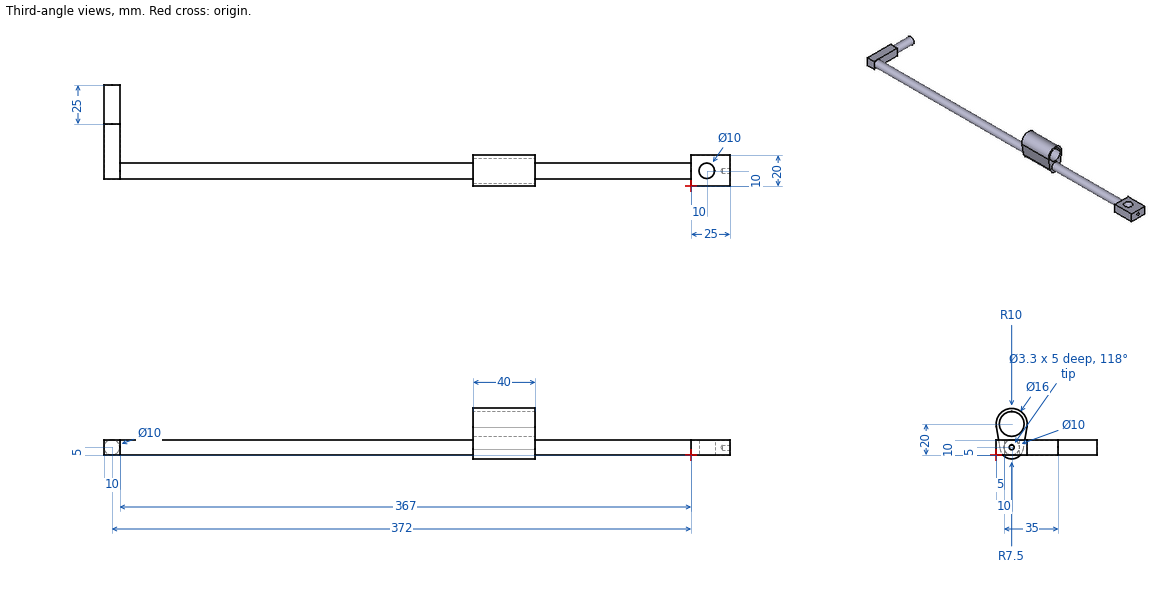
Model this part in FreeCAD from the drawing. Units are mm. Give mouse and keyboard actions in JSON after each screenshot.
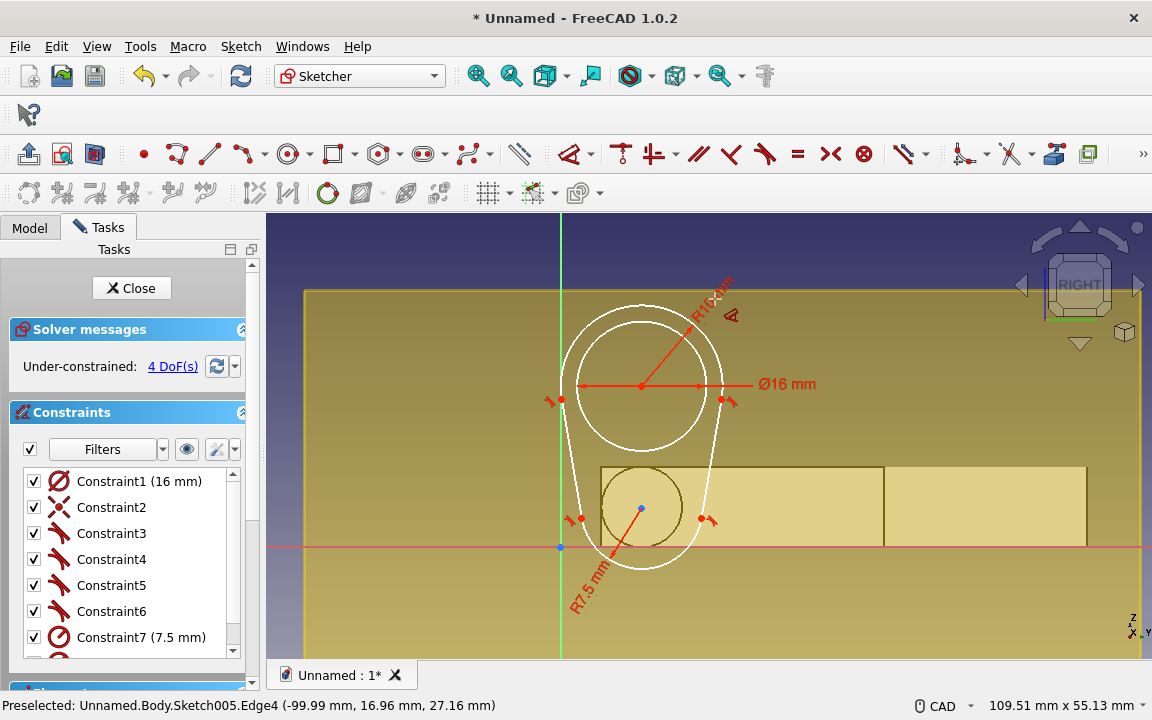
{"action": "left_click", "coordinate": [642, 508]}
{"action": "left_click", "coordinate": [527, 528]}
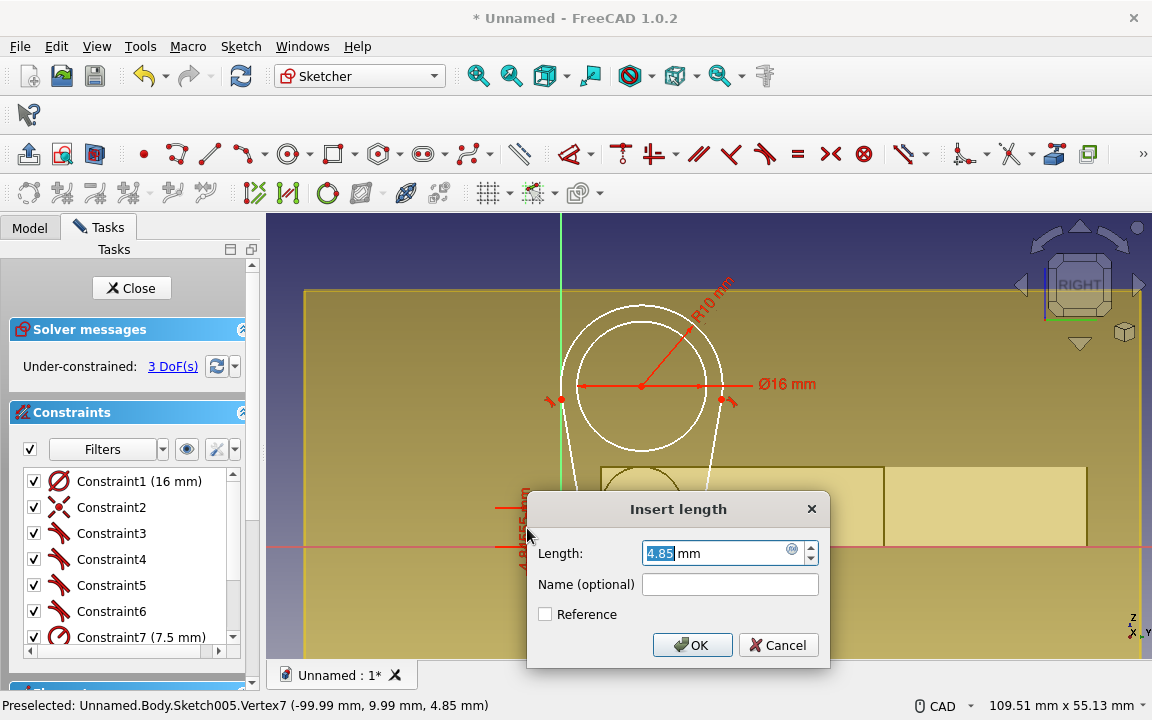
{"action": "type", "text": "5"}
{"action": "key", "text": "Return"}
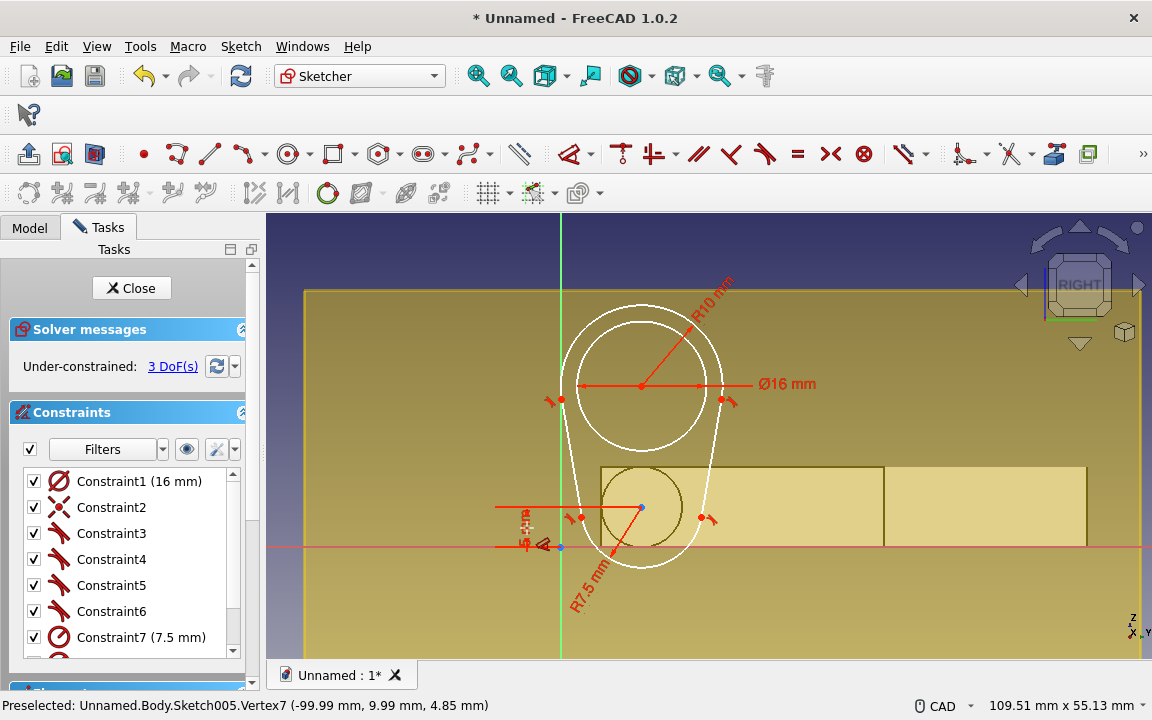
{"action": "left_click", "coordinate": [642, 386]}
{"action": "left_click", "coordinate": [620, 352]}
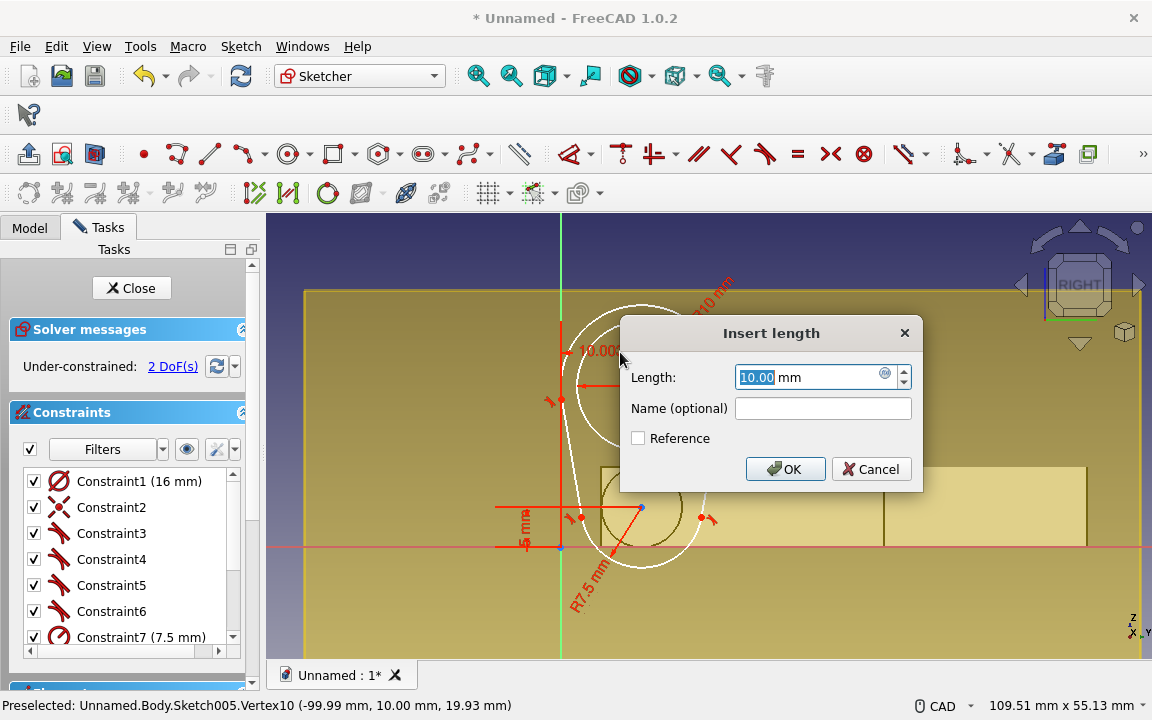
{"action": "type", "text": "10"}
{"action": "key", "text": "Return"}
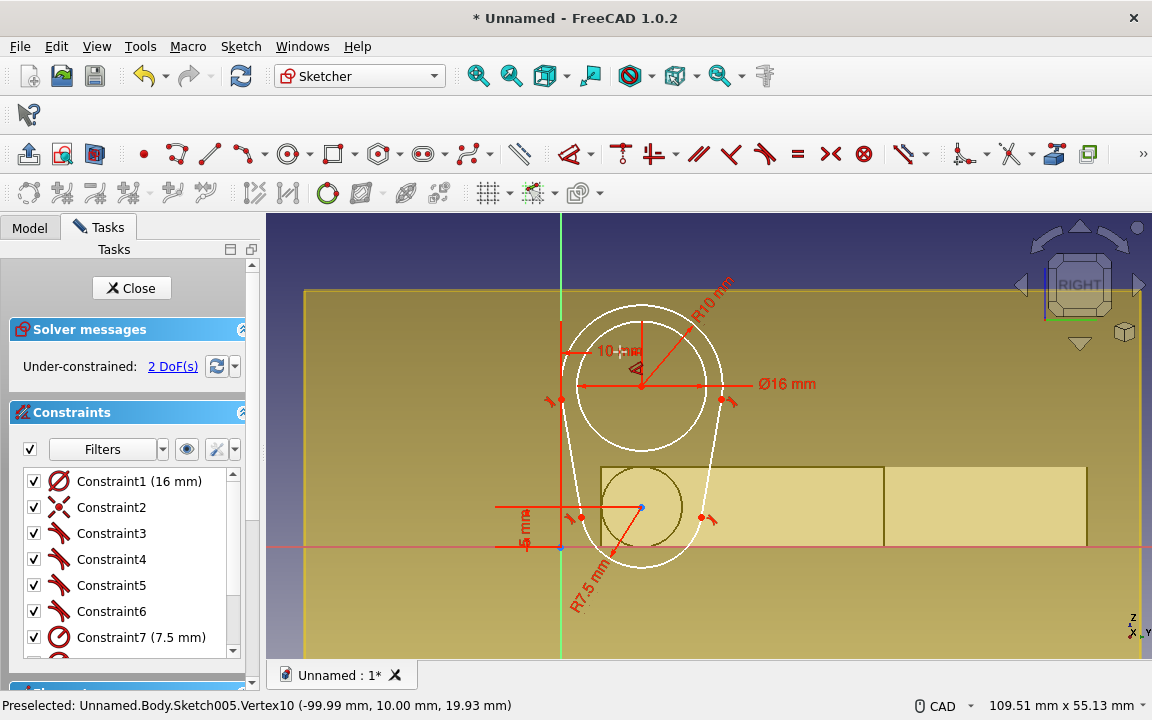
{"action": "left_click", "coordinate": [642, 386]}
{"action": "left_click", "coordinate": [527, 467]}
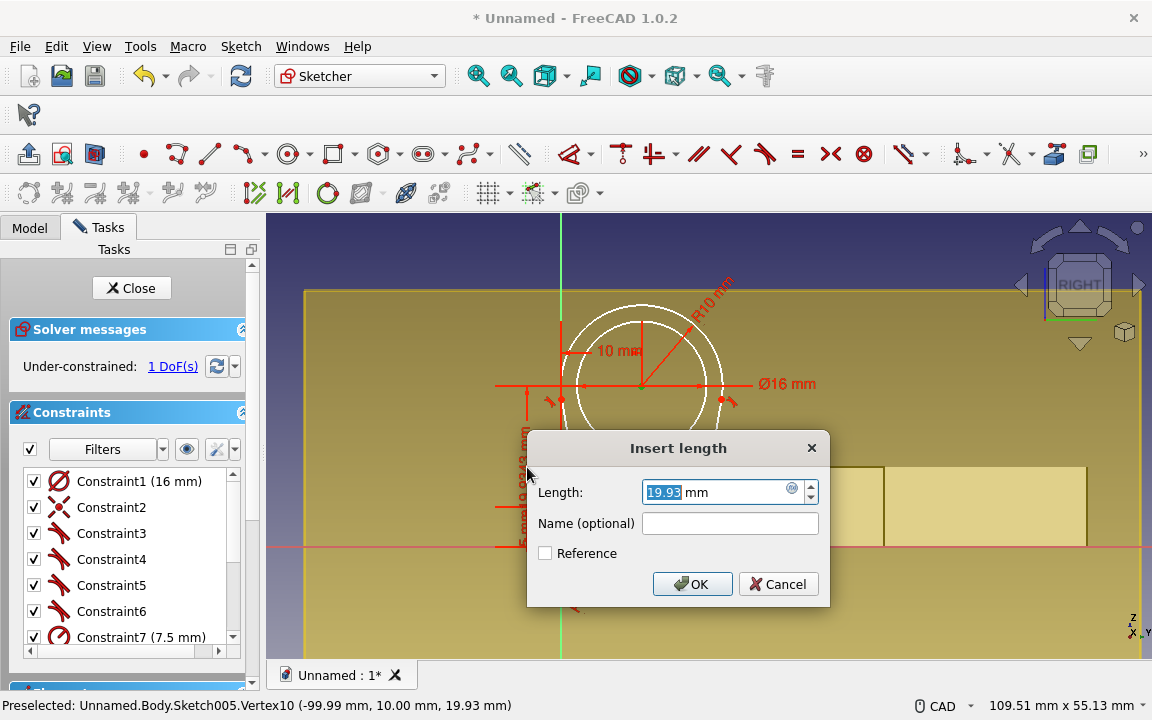
{"action": "type", "text": "20"}
{"action": "key", "text": "Return"}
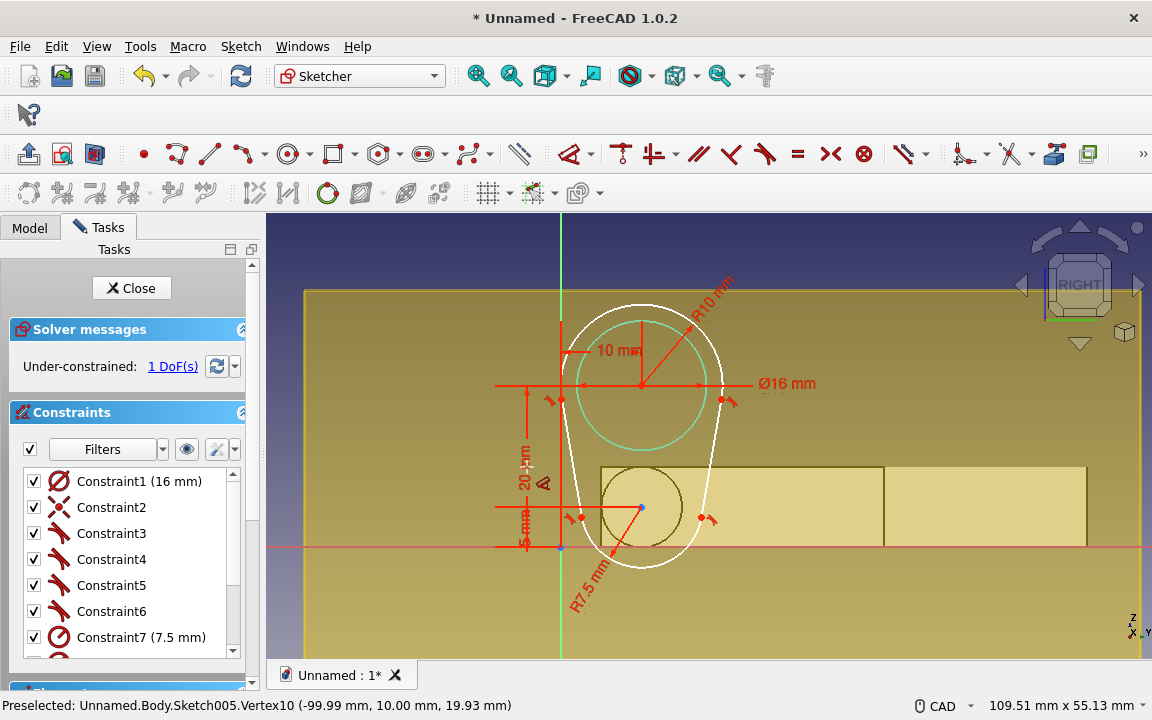
{"action": "left_click", "coordinate": [642, 507]}
{"action": "left_click", "coordinate": [601, 473]}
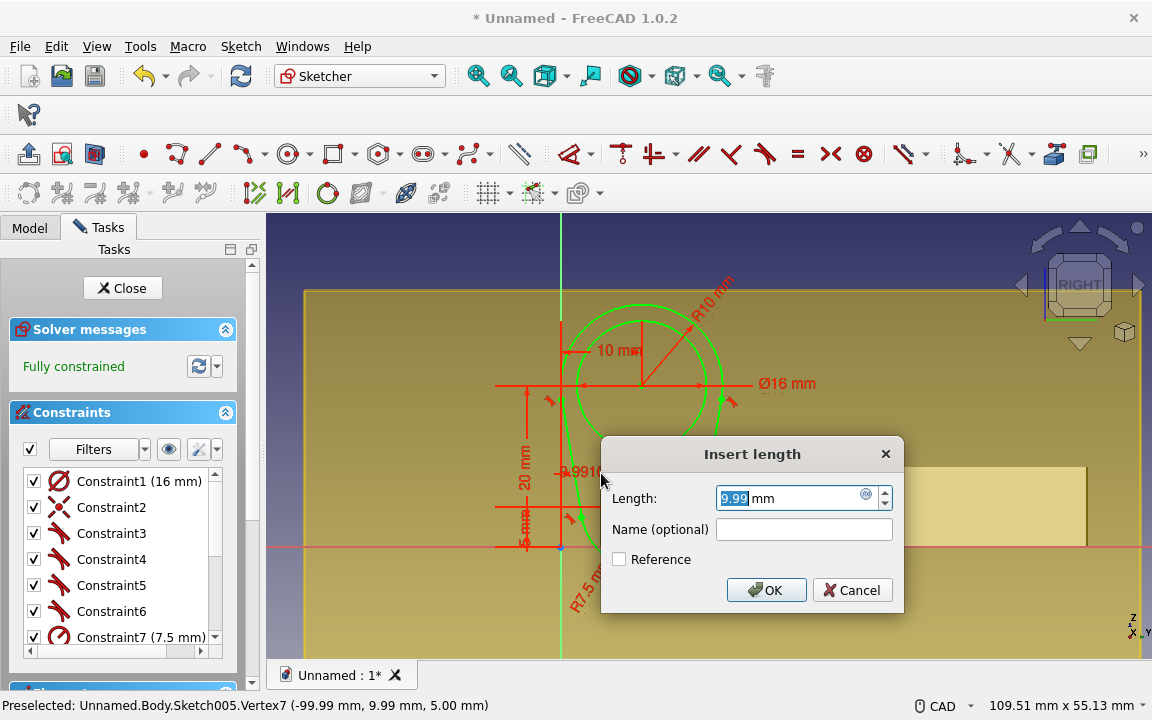
{"action": "type", "text": "10"}
{"action": "key", "text": "Return"}
{"action": "key", "text": "Escape"}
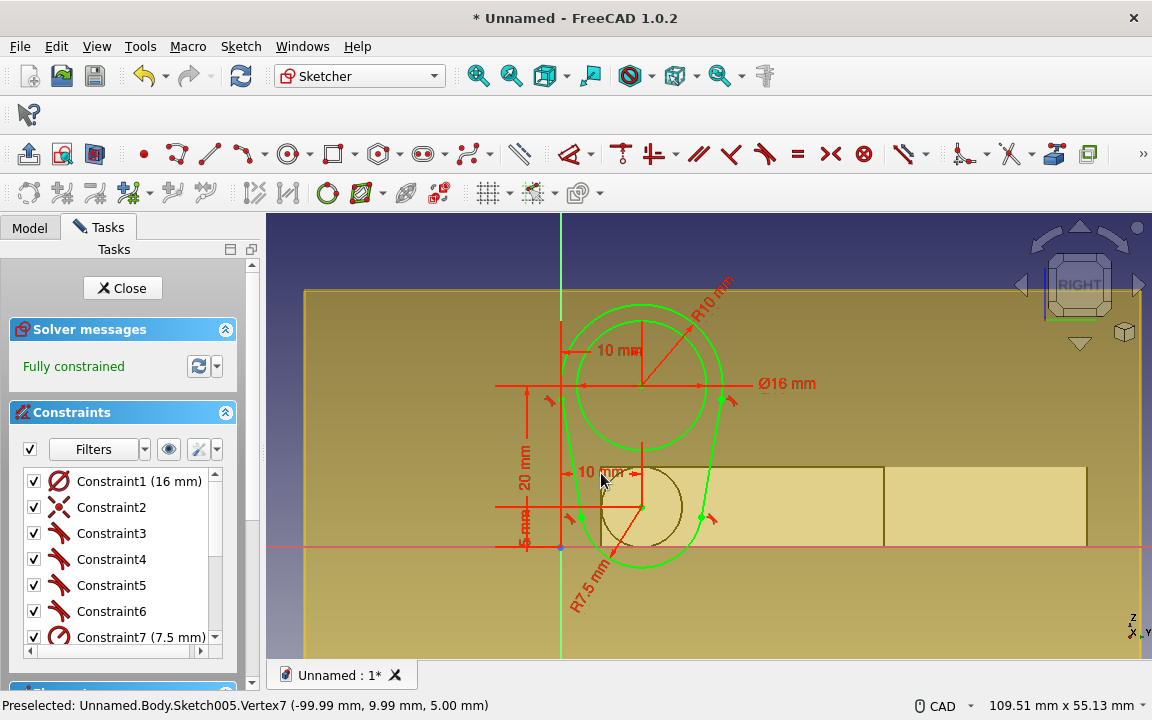
{"action": "left_click", "coordinate": [123, 288]}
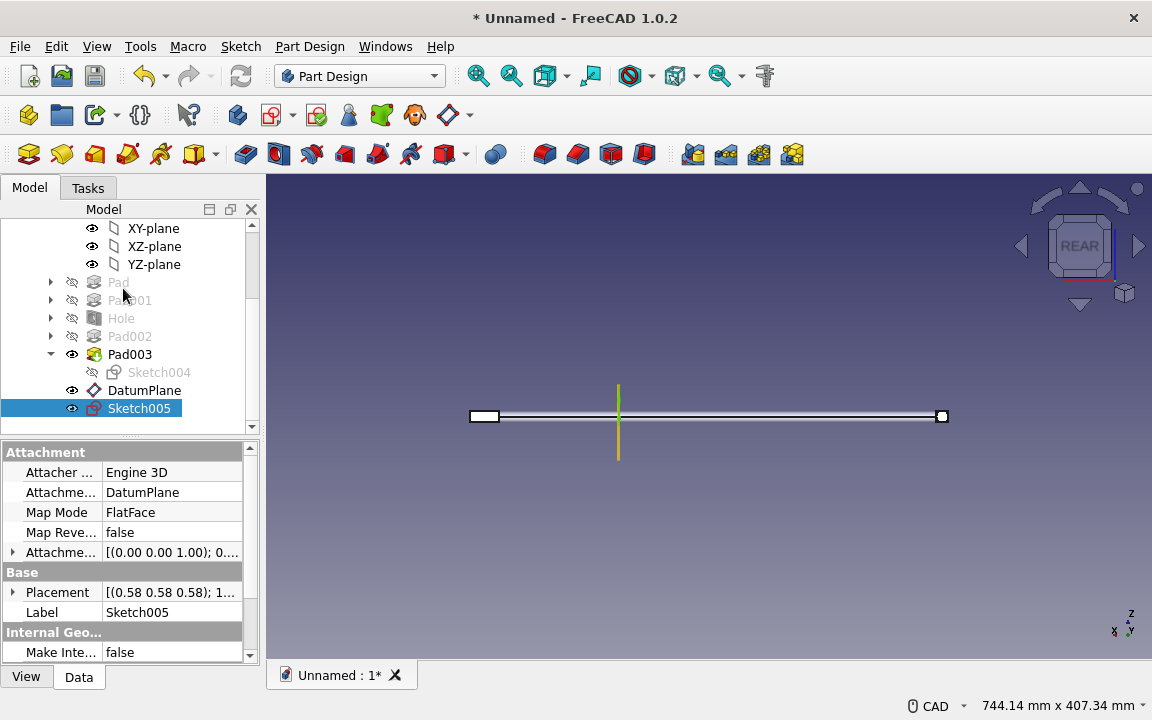
{"action": "left_click", "coordinate": [29, 154]}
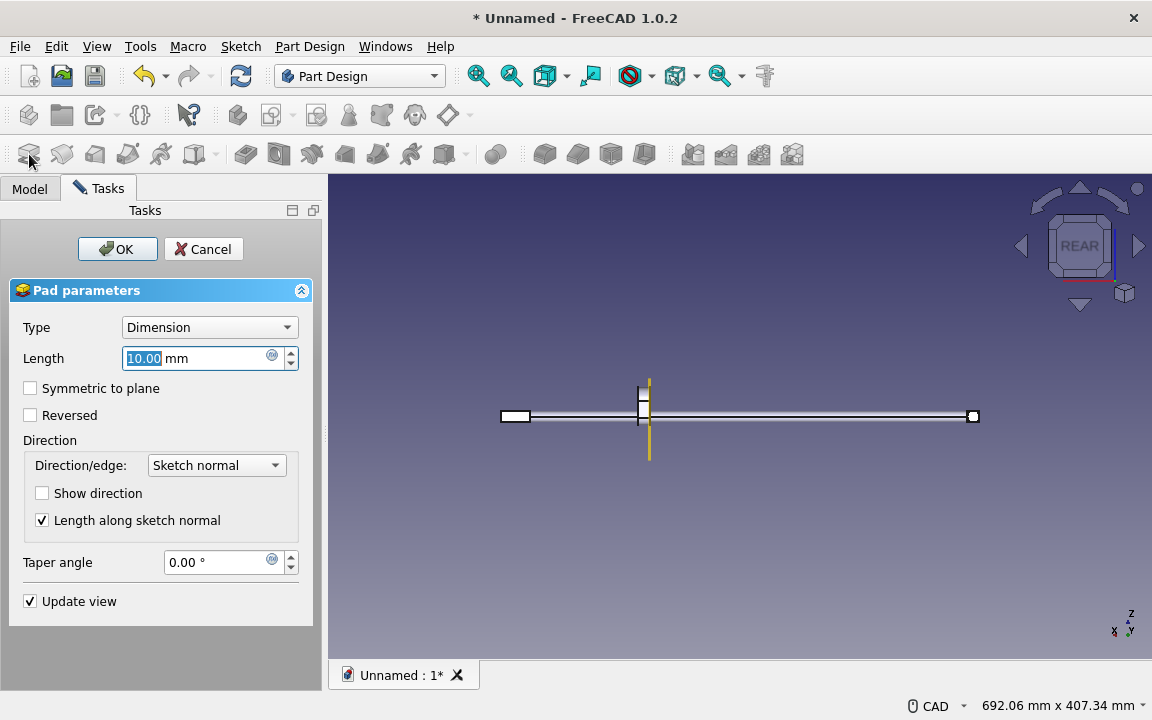
{"action": "type", "text": "40"}
{"action": "key", "text": "Tab"}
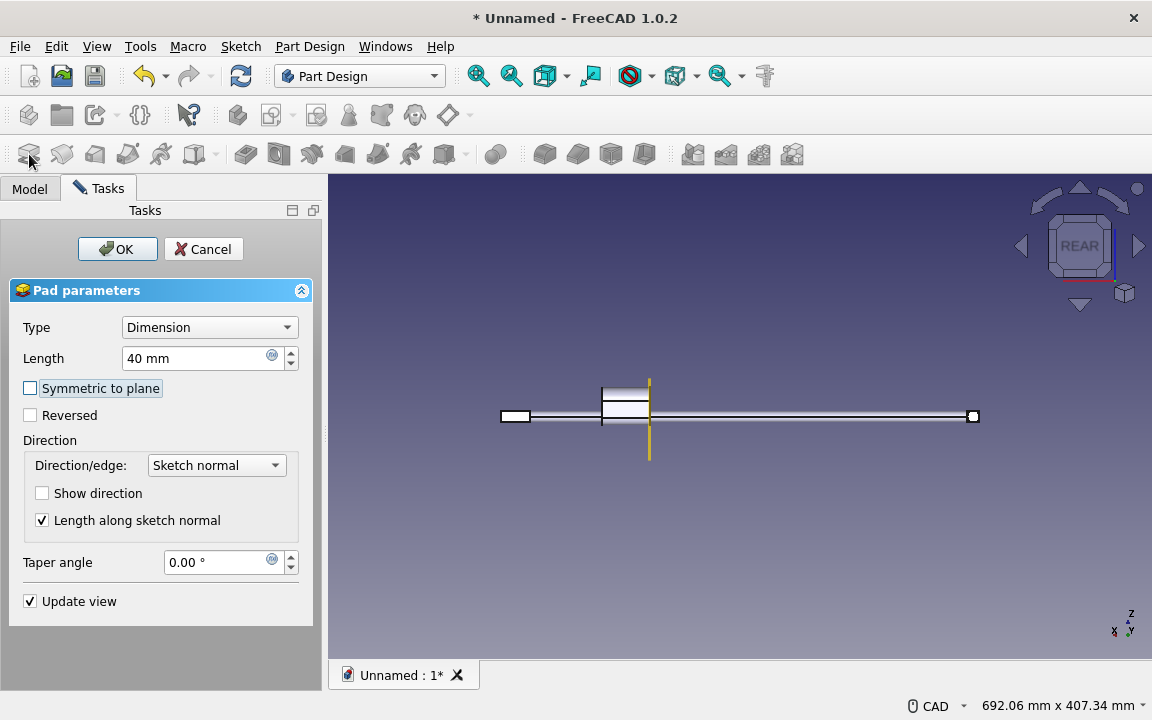
{"action": "left_click", "coordinate": [31, 415]}